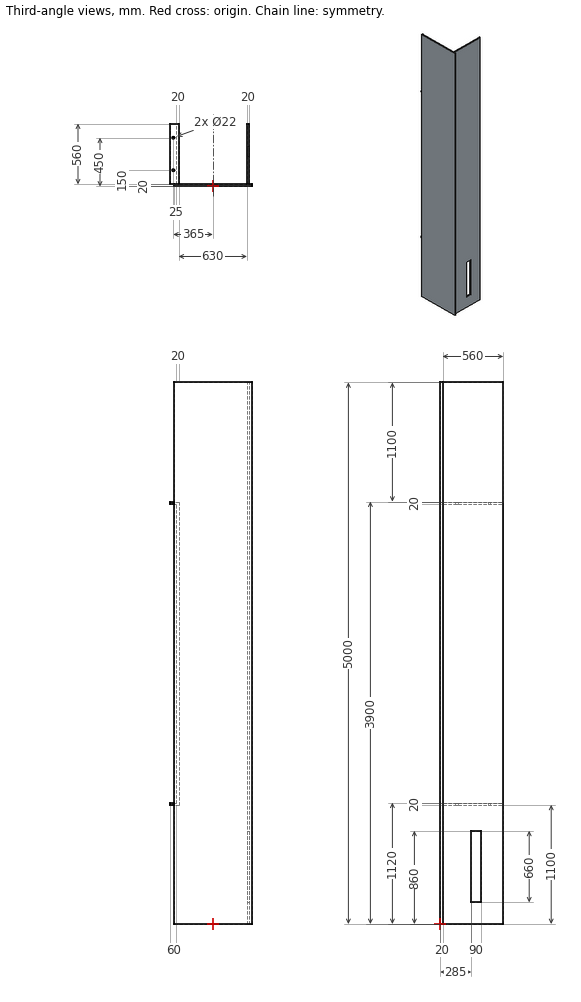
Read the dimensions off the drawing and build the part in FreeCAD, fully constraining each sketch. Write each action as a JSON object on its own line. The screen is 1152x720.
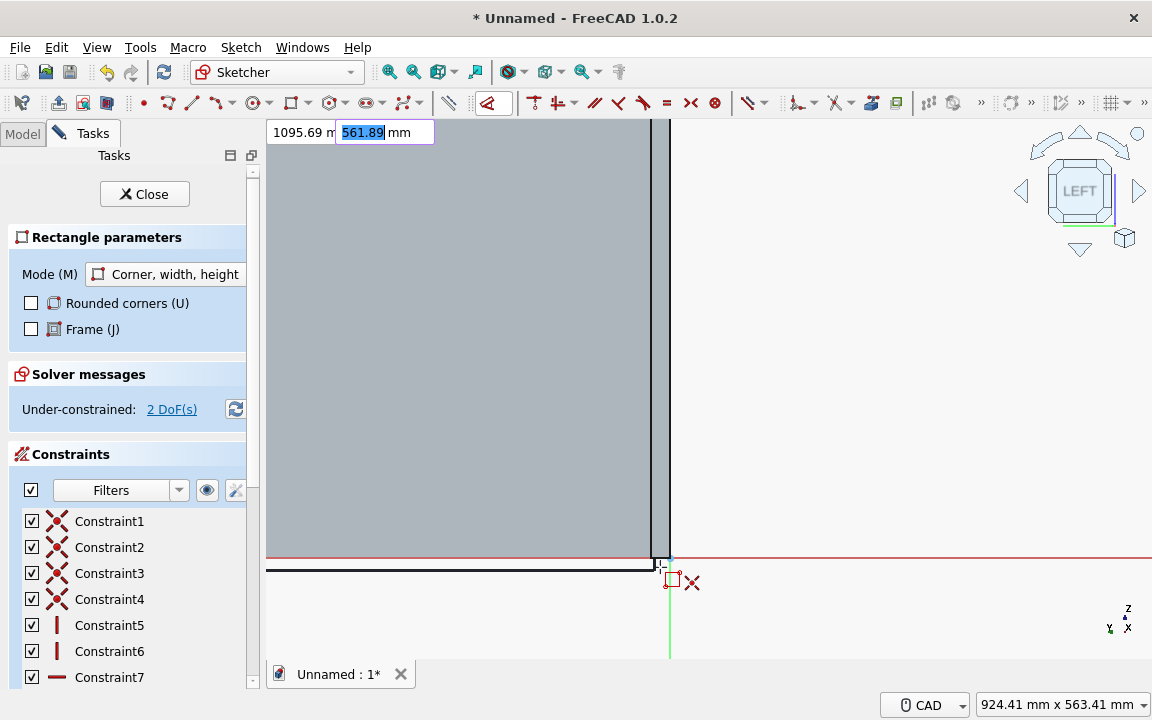
{"action": "left_click", "coordinate": [651, 558]}
{"action": "key", "text": "Escape"}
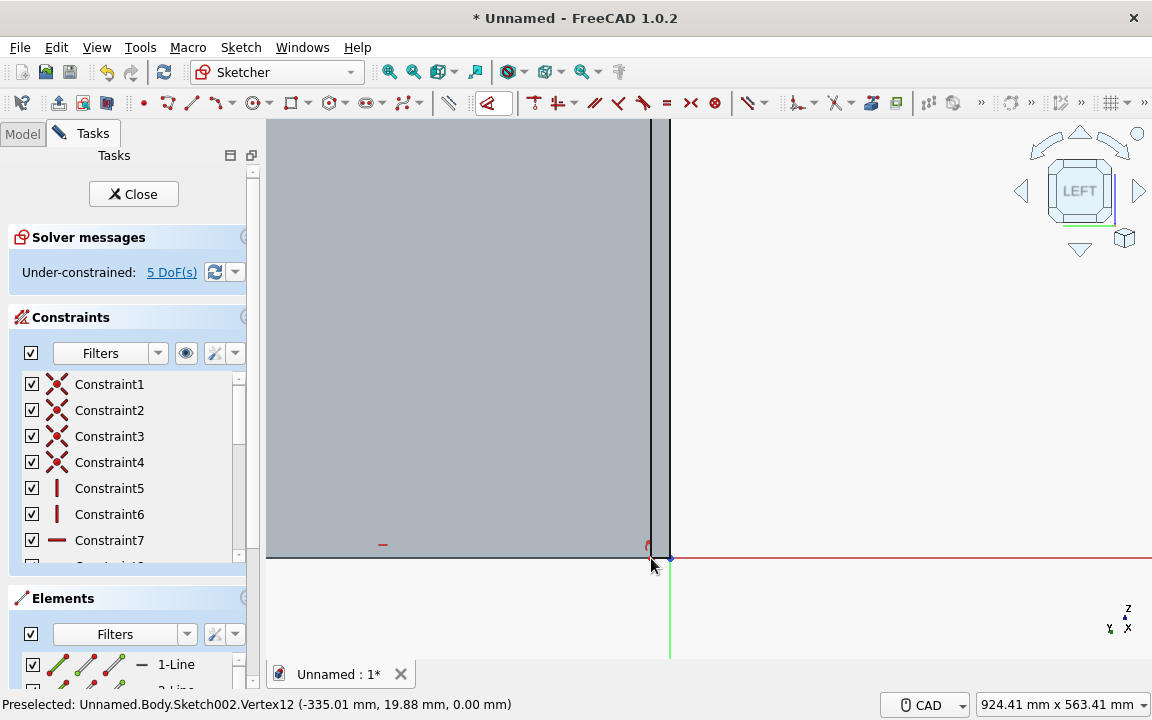
{"action": "scroll", "coordinate": [660, 568], "scroll_direction": "down", "scroll_amount": 13}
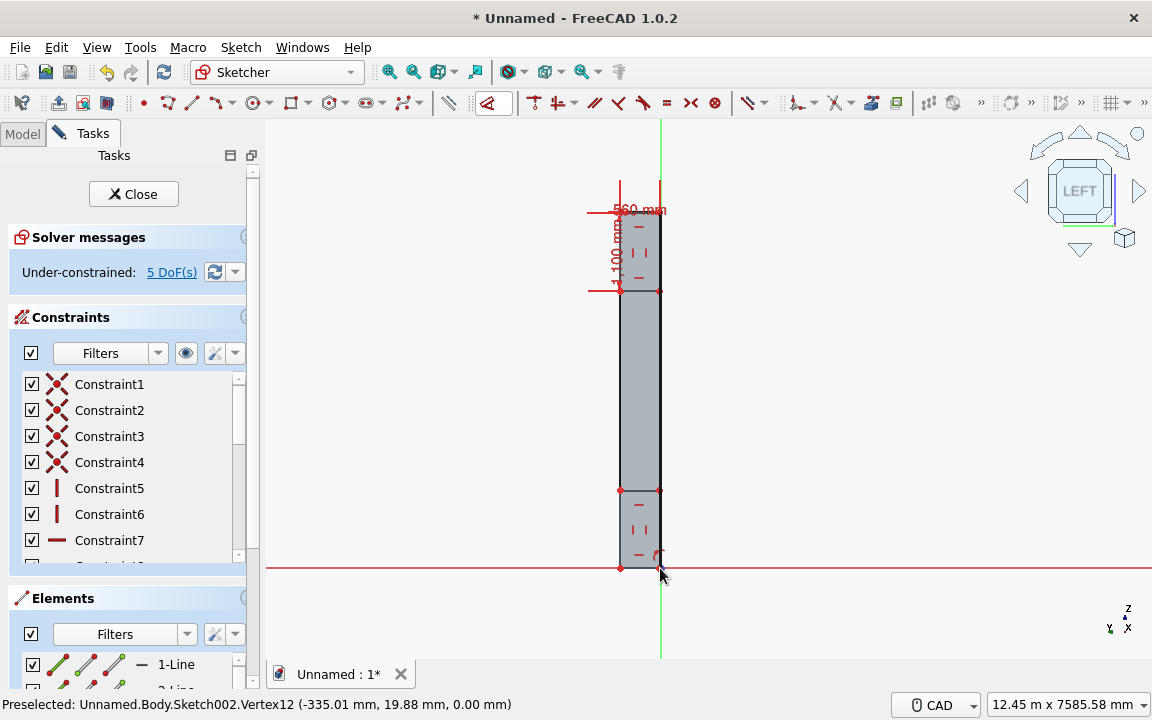
{"action": "left_click", "coordinate": [648, 568]}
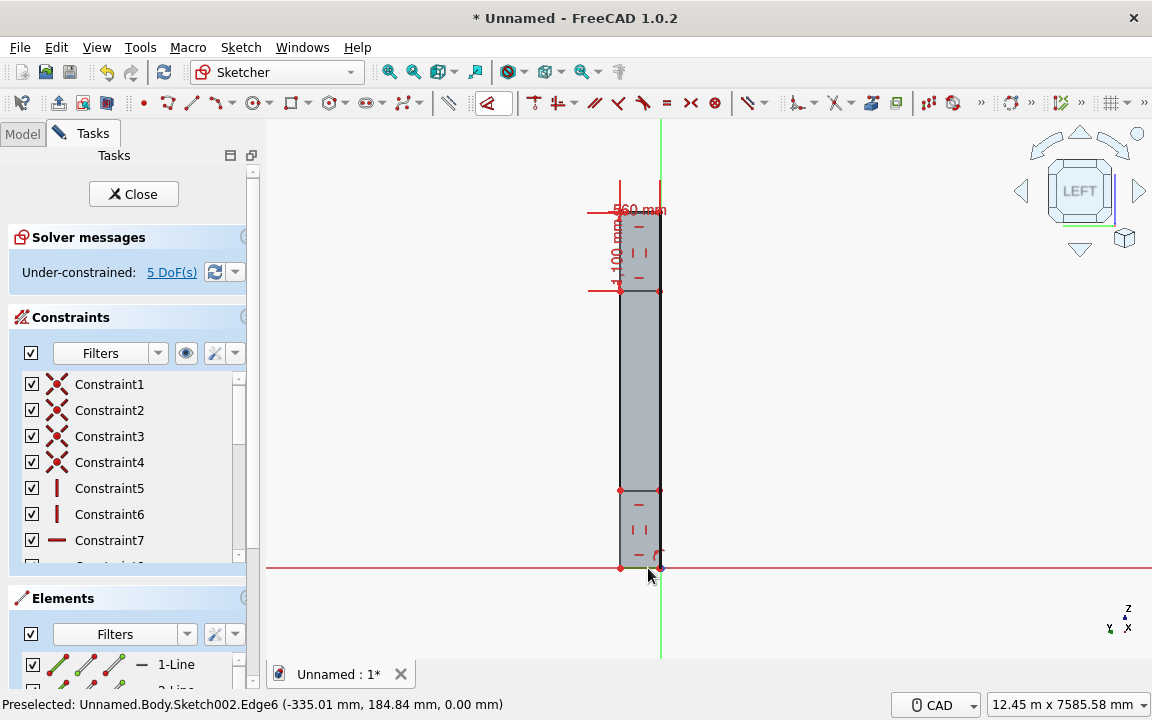
{"action": "left_click", "coordinate": [506, 104]}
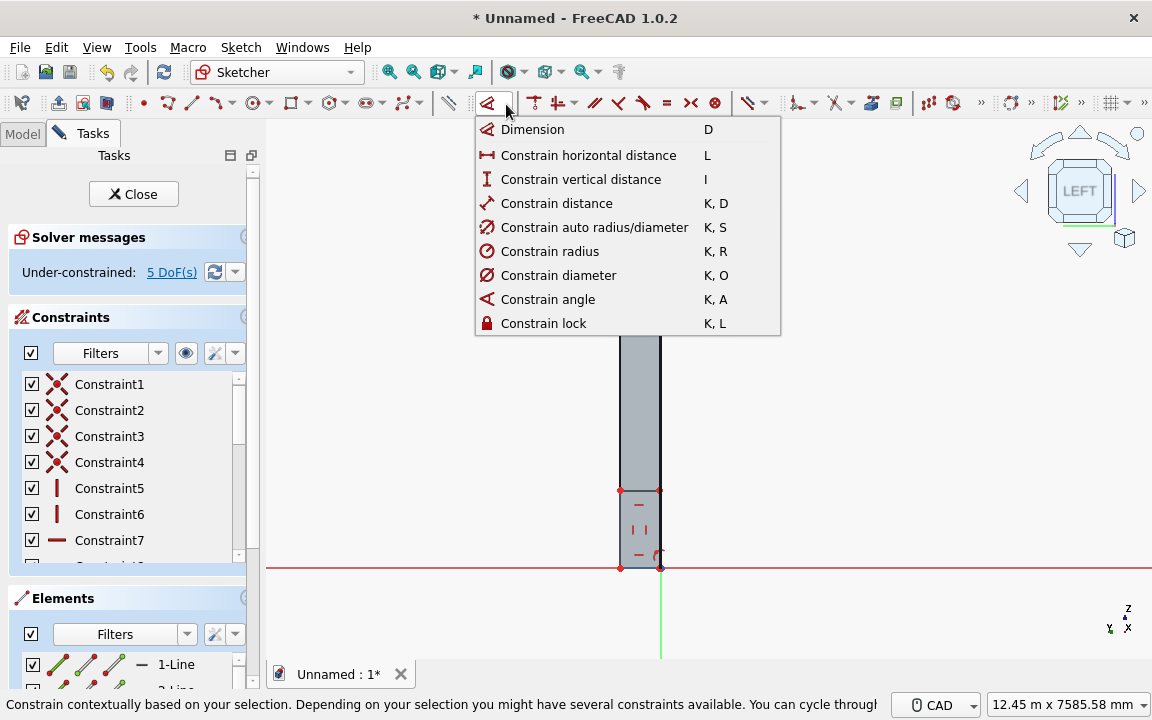
{"action": "left_click", "coordinate": [628, 155]}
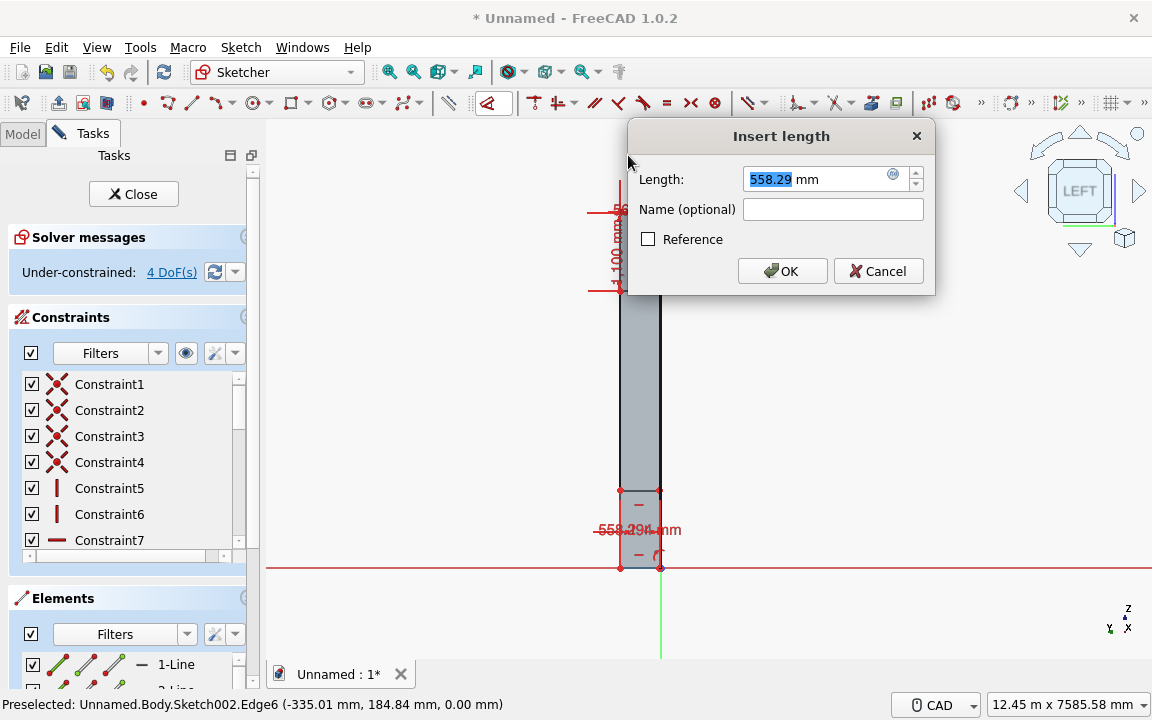
{"action": "type", "text": "560"}
{"action": "key", "text": "Return"}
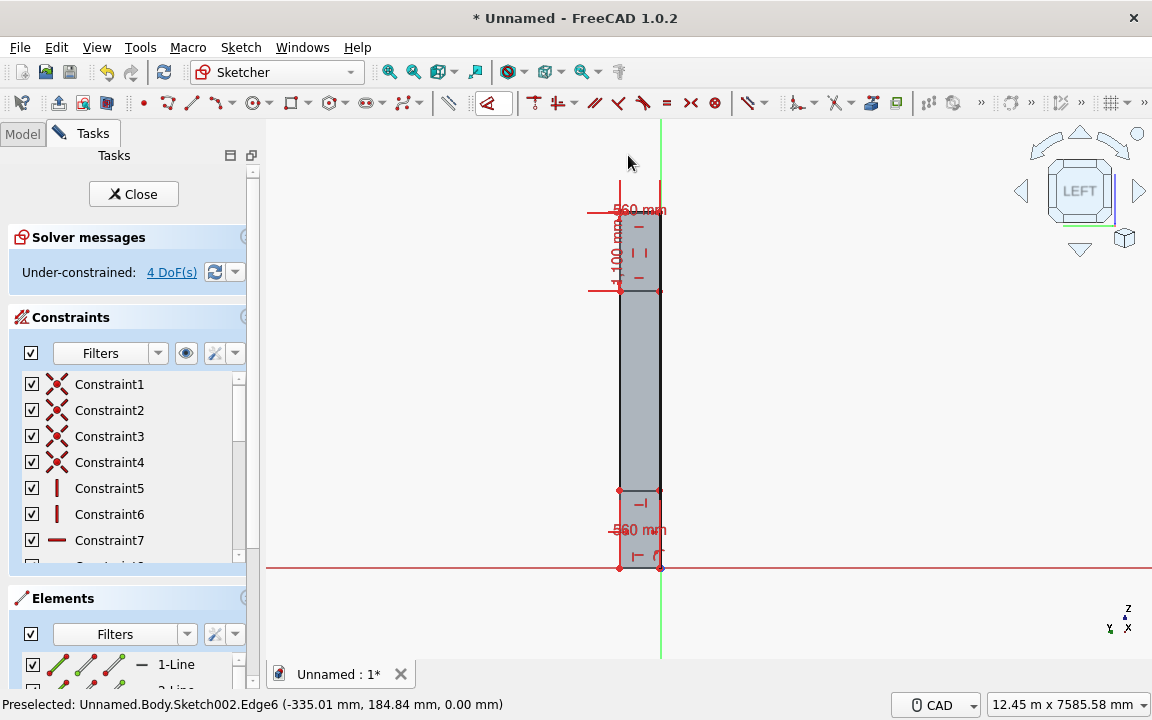
{"action": "scroll", "coordinate": [660, 291], "scroll_direction": "up", "scroll_amount": 17}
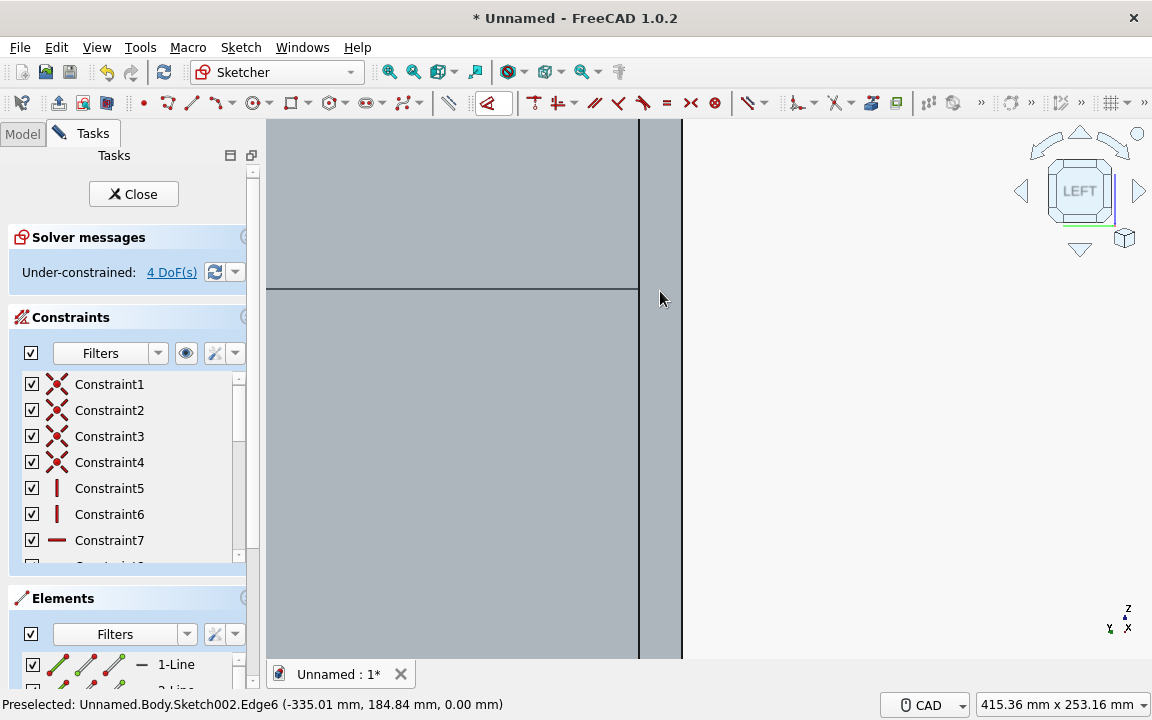
{"action": "left_click", "coordinate": [643, 289]}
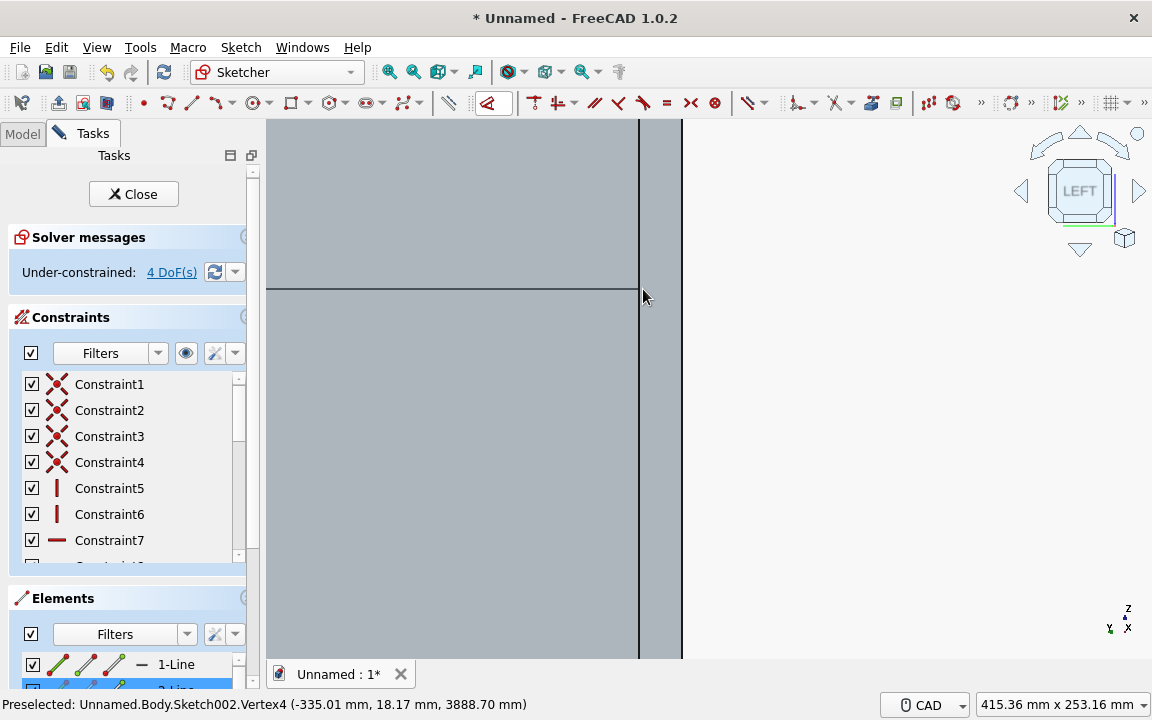
{"action": "left_click", "coordinate": [506, 104]}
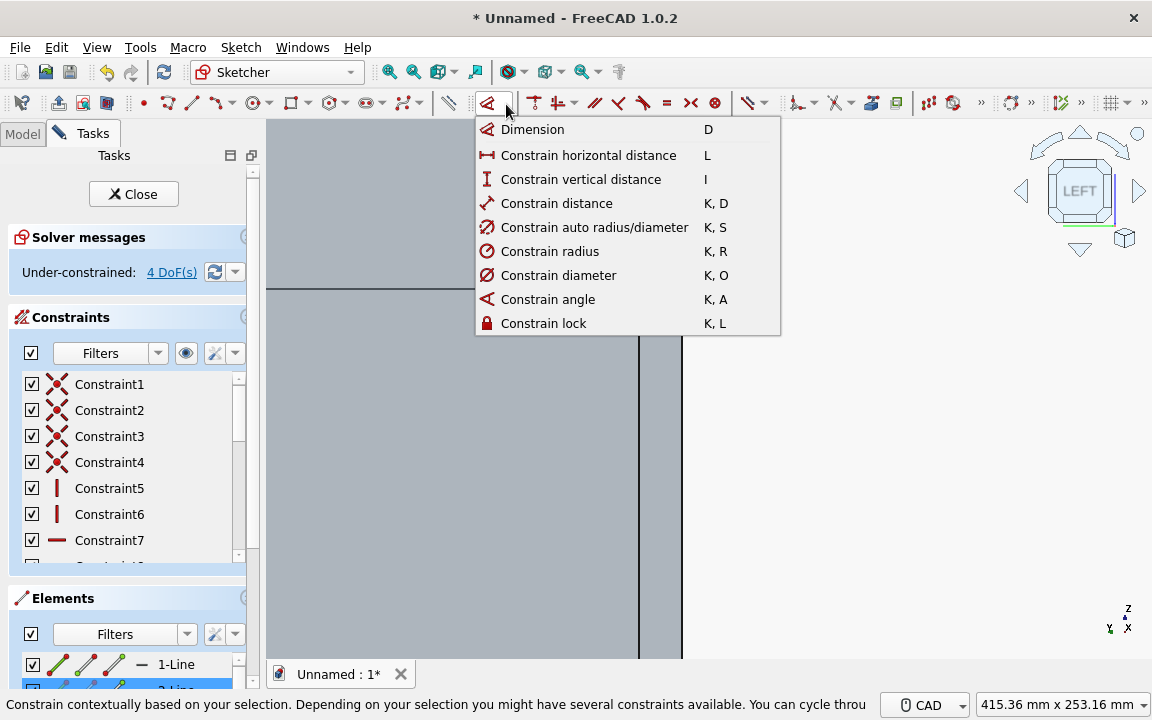
{"action": "left_click", "coordinate": [628, 155]}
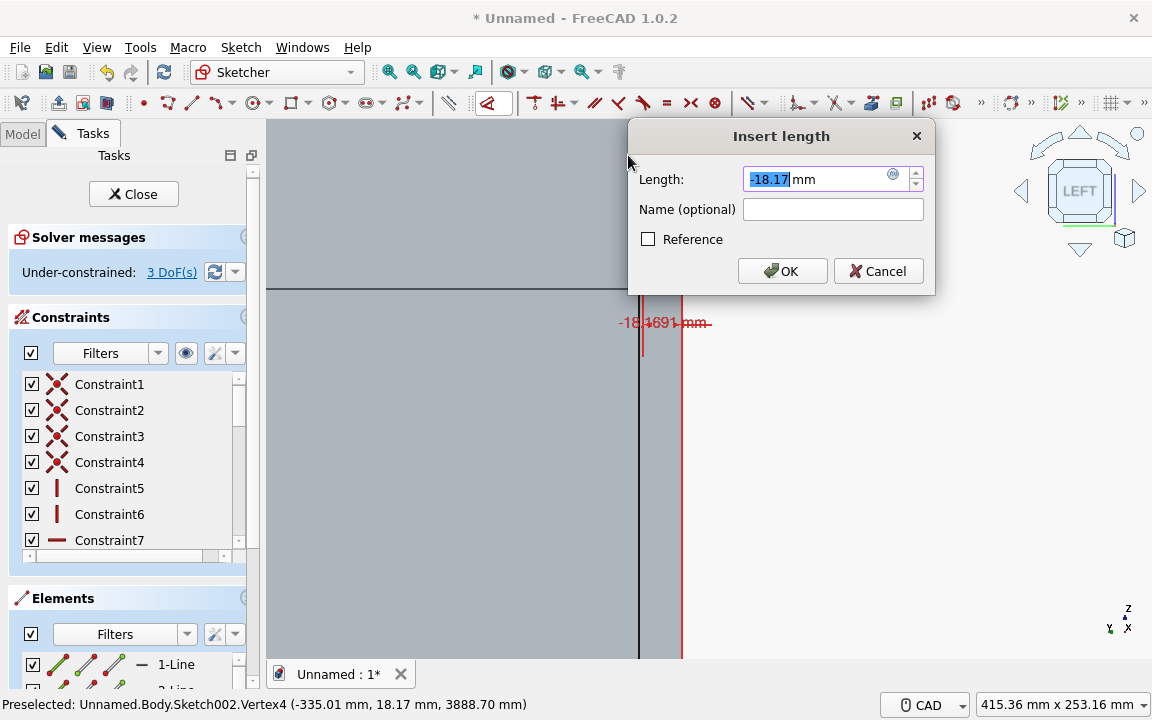
{"action": "type", "text": "-20"}
{"action": "key", "text": "Return"}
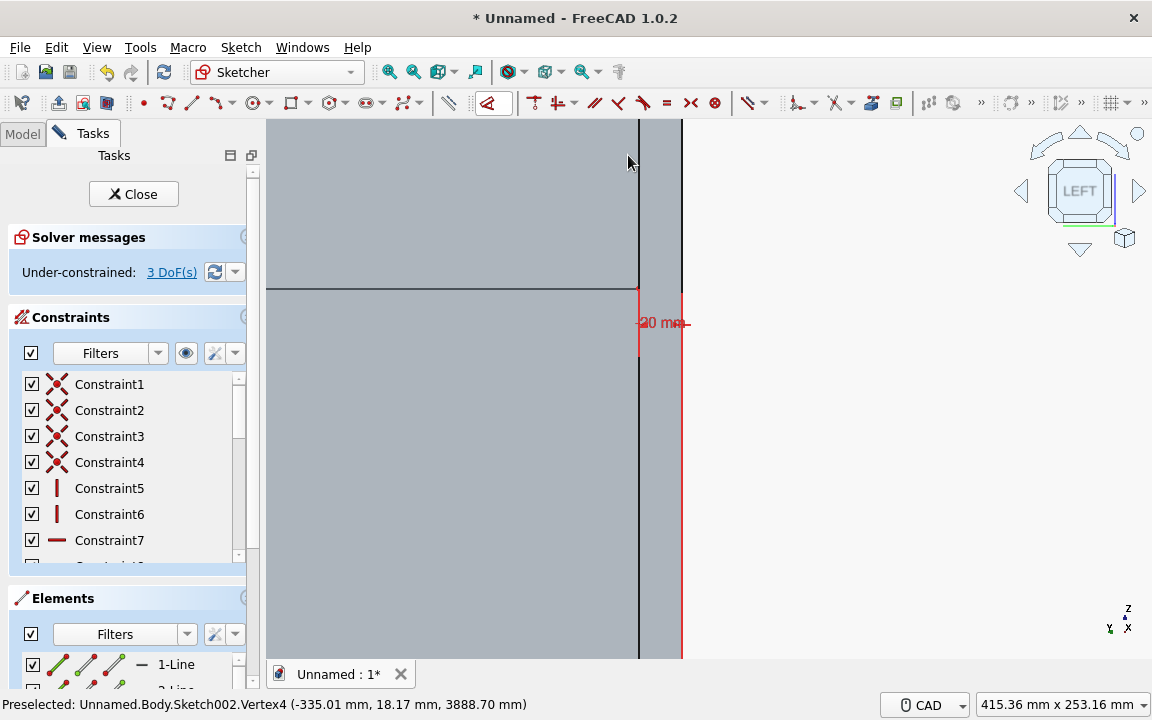
{"action": "scroll", "coordinate": [660, 290], "scroll_direction": "down", "scroll_amount": 17}